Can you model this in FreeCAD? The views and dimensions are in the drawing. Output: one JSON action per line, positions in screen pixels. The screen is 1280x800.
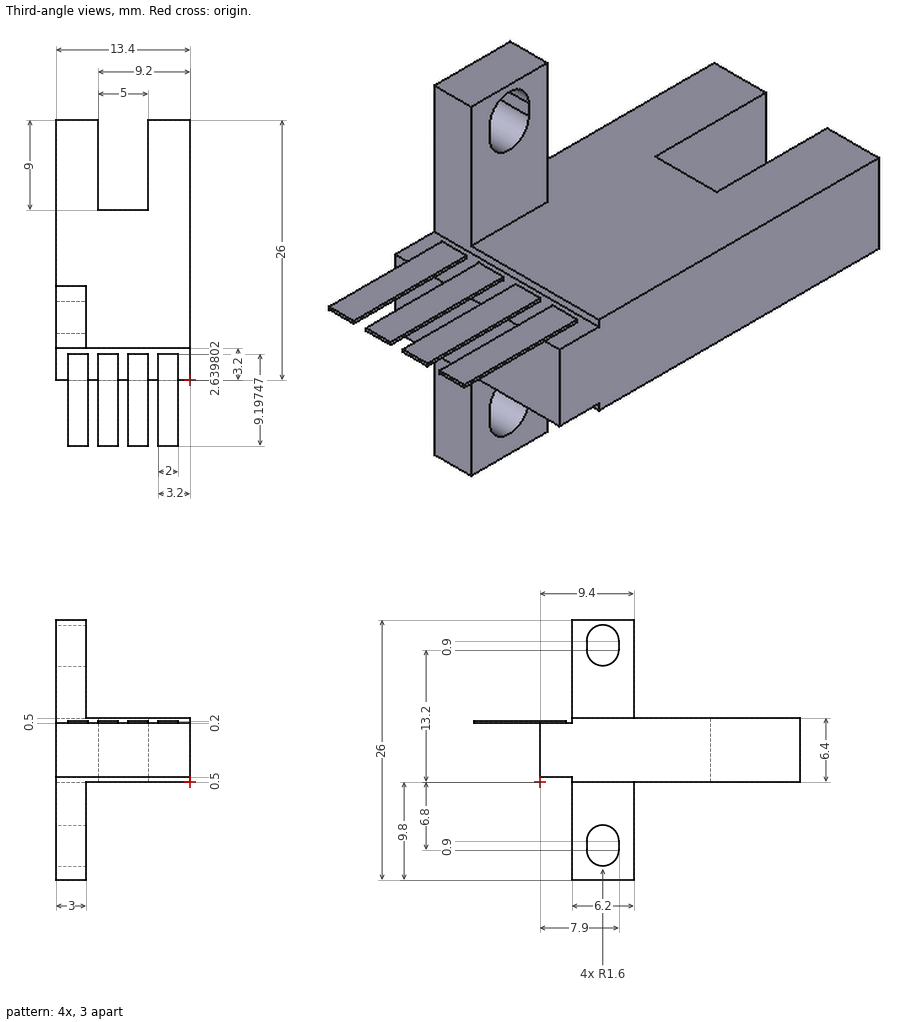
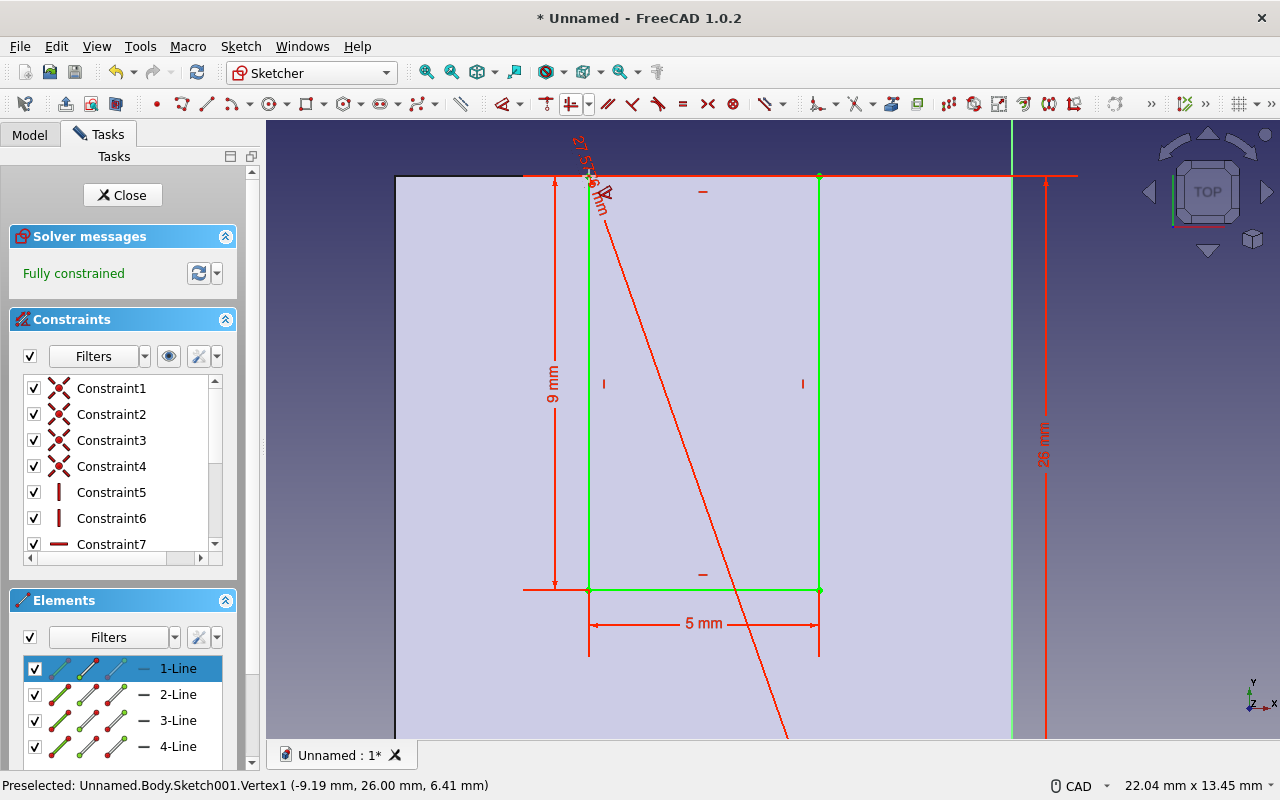
{"action": "key", "text": "Escape"}
{"action": "key", "text": "Escape"}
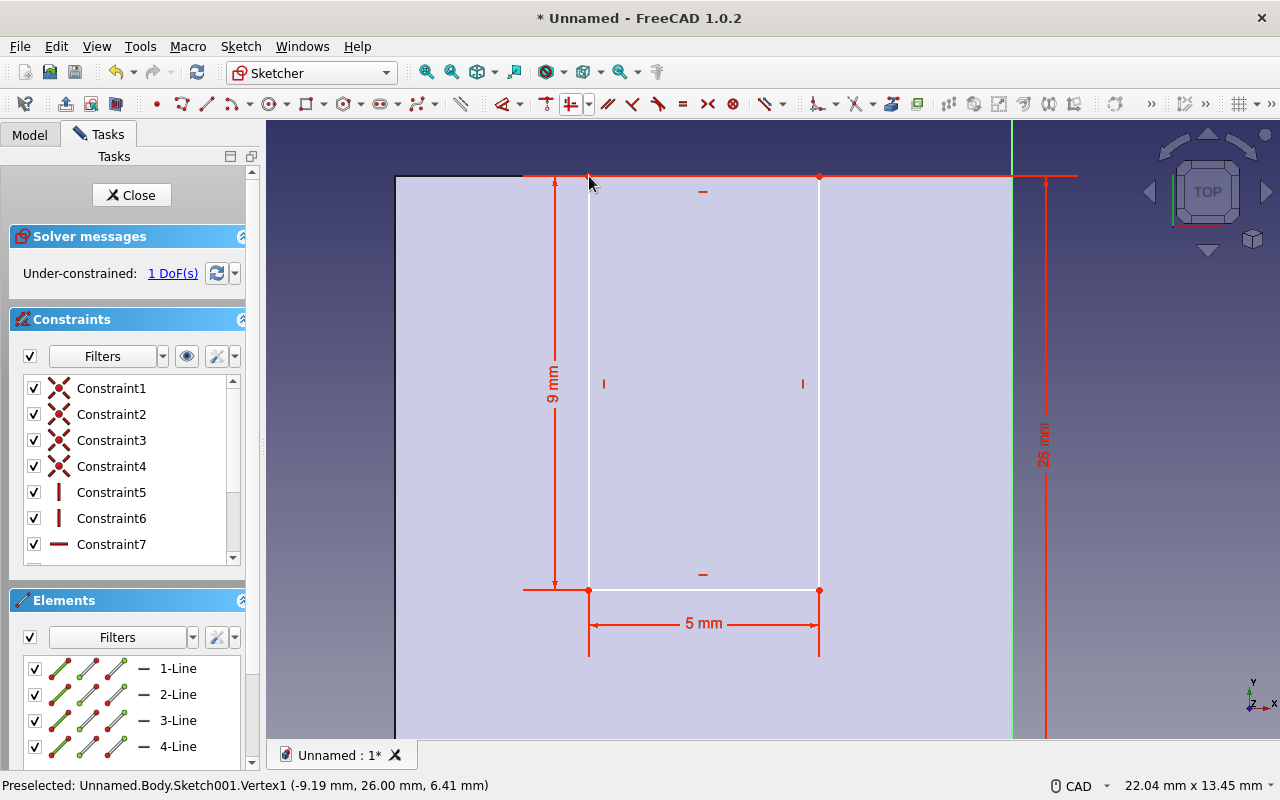
{"action": "left_click", "coordinate": [589, 176]}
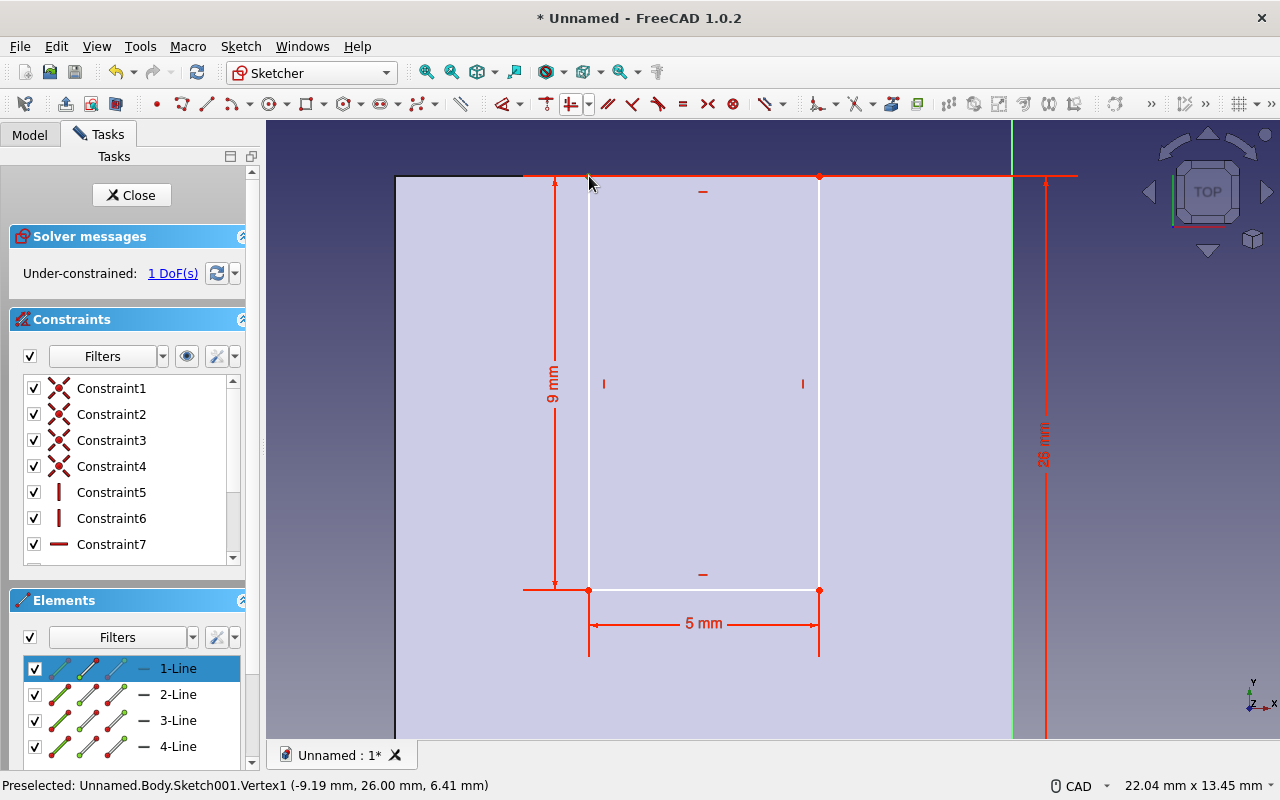
{"action": "key", "text": "l"}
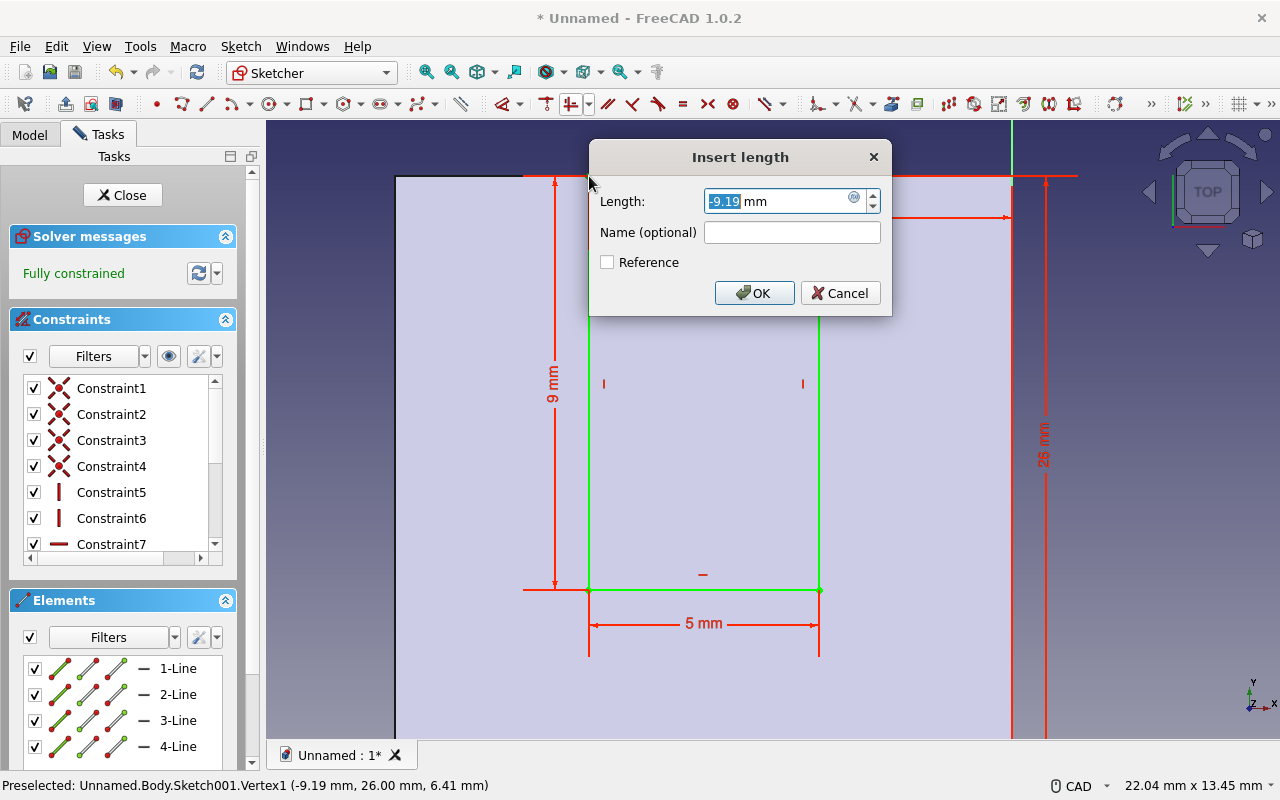
{"action": "type", "text": "-9.2"}
{"action": "key", "text": "Return"}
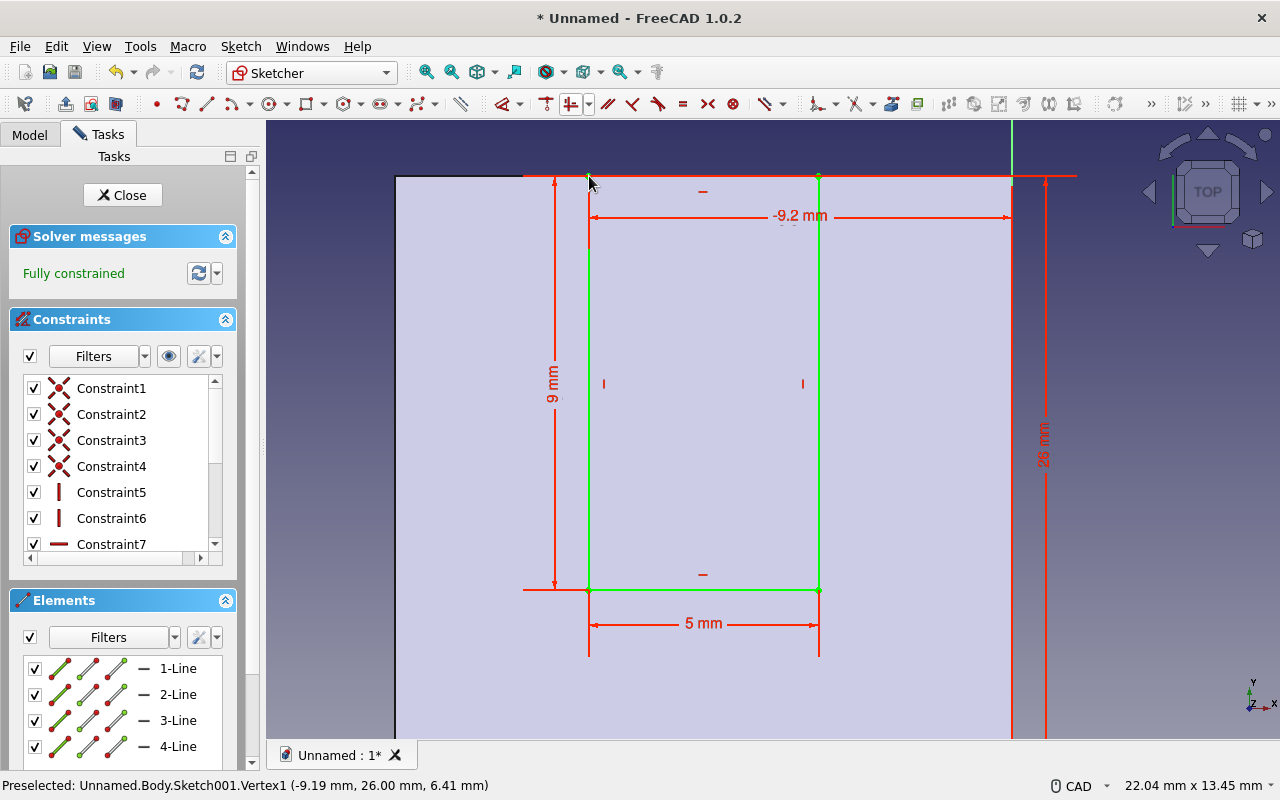
{"action": "left_click", "coordinate": [123, 195]}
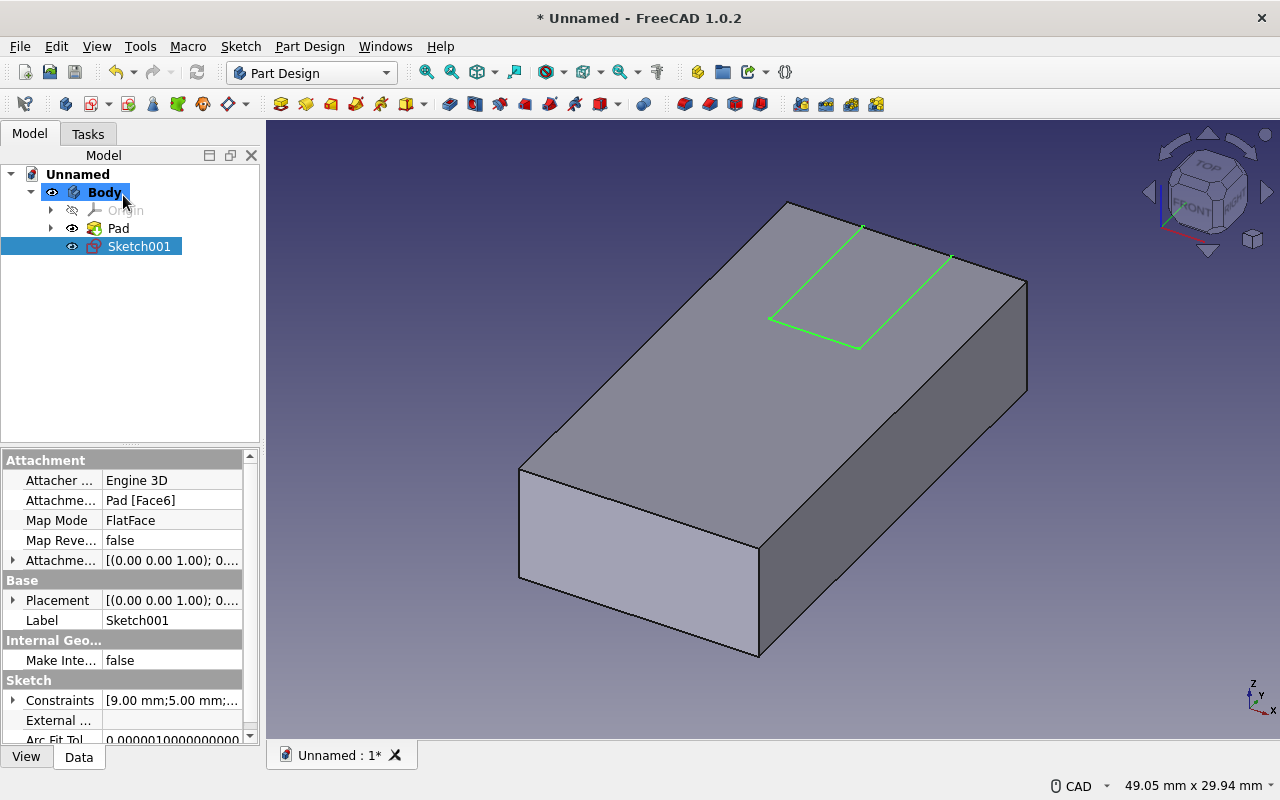
{"action": "left_click", "coordinate": [450, 104]}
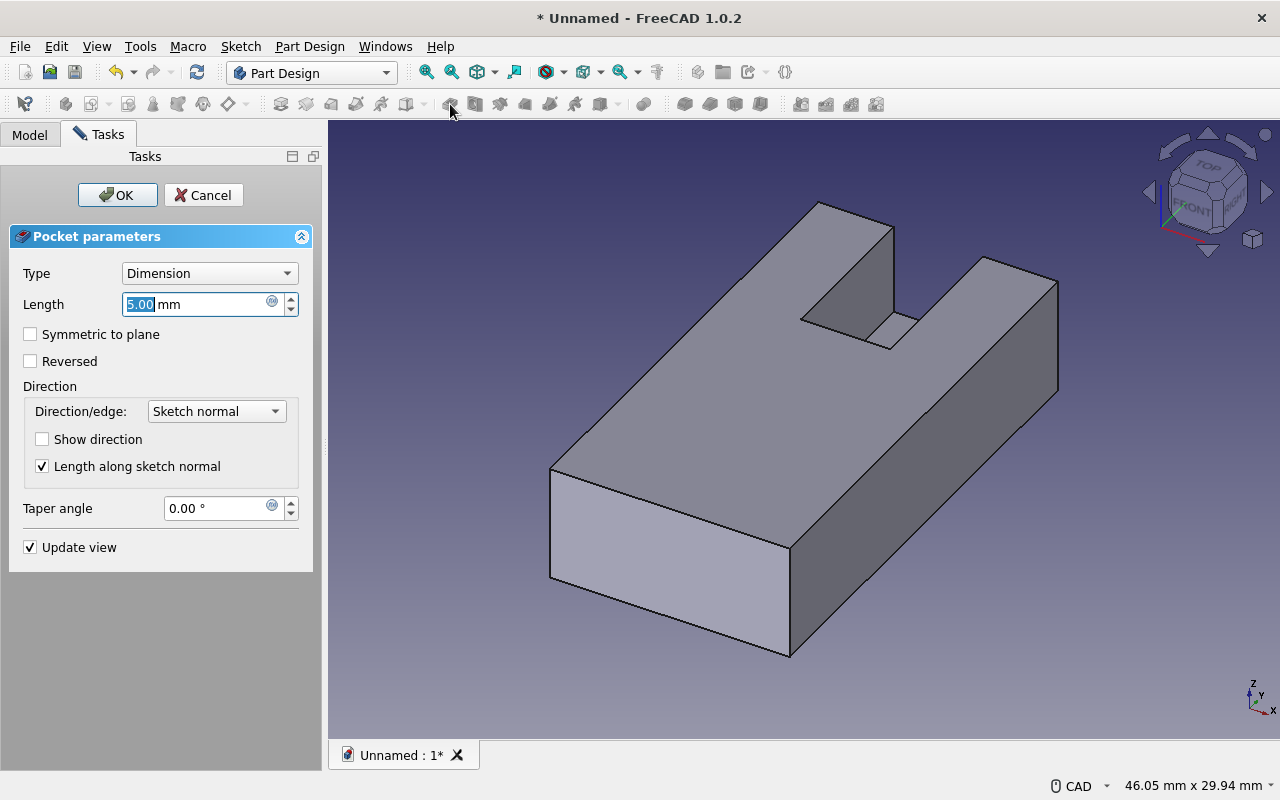
{"action": "left_click", "coordinate": [210, 274]}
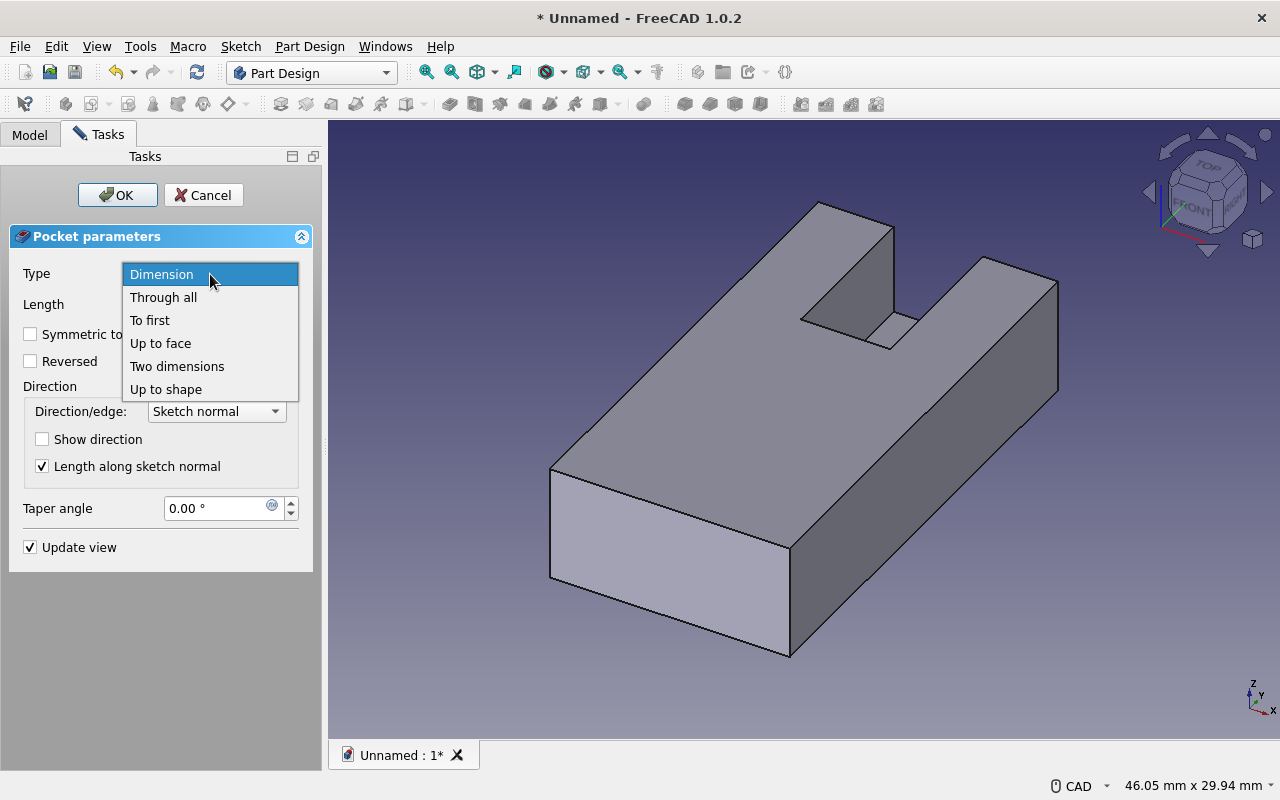
{"action": "left_click", "coordinate": [208, 298]}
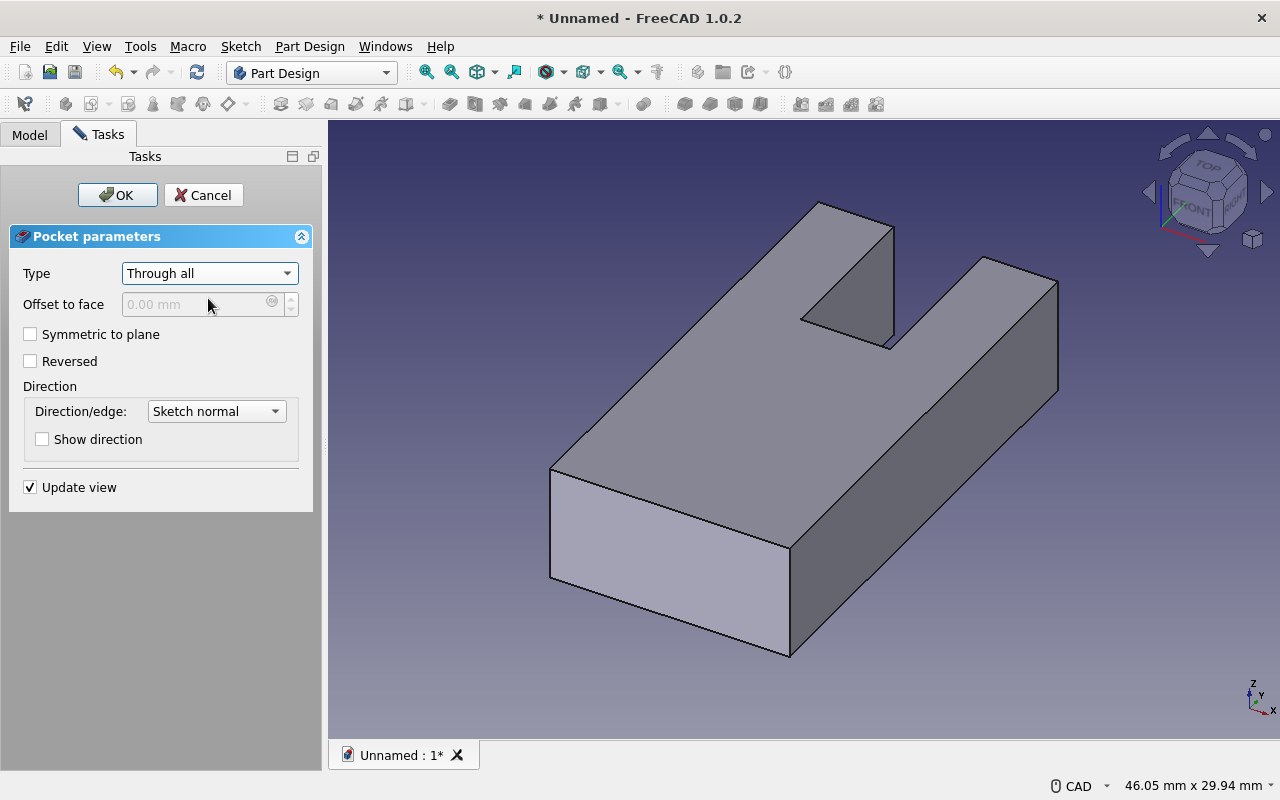
{"action": "left_click", "coordinate": [118, 195]}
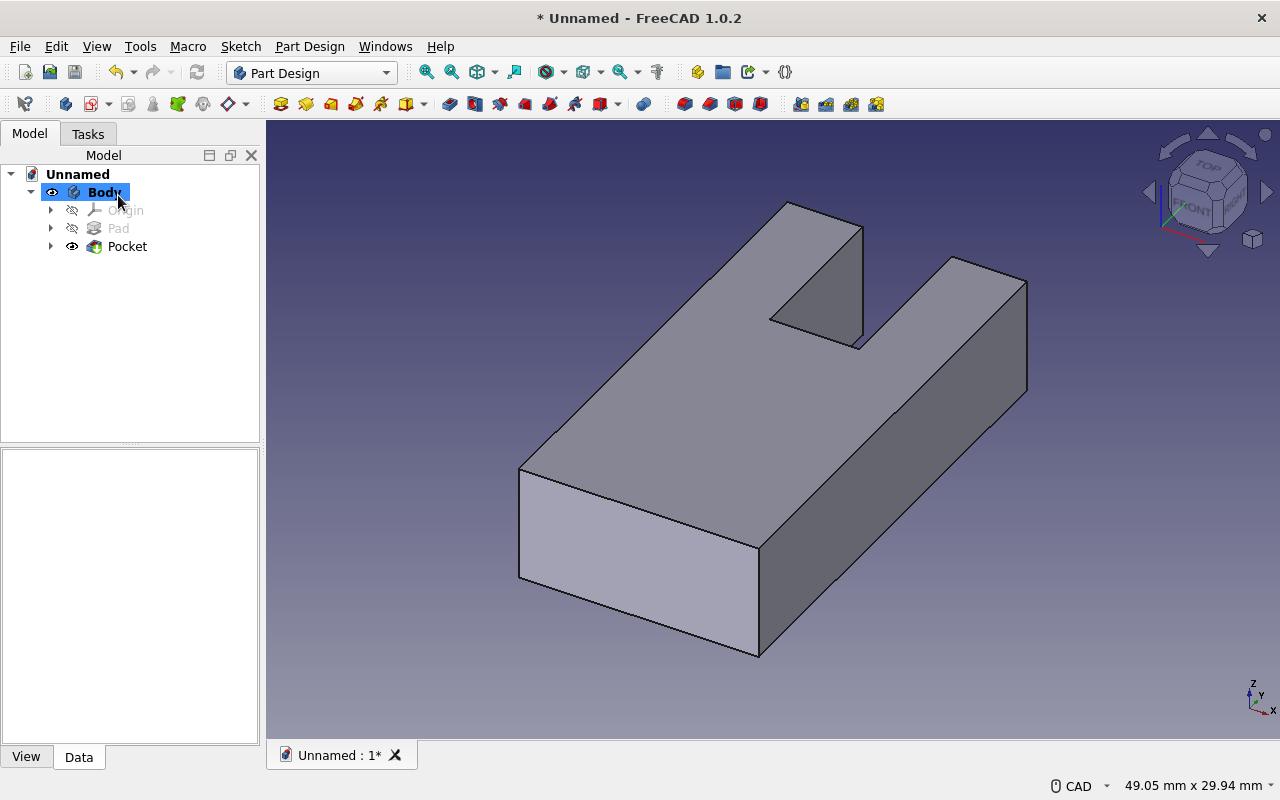
{"action": "key", "text": "6"}